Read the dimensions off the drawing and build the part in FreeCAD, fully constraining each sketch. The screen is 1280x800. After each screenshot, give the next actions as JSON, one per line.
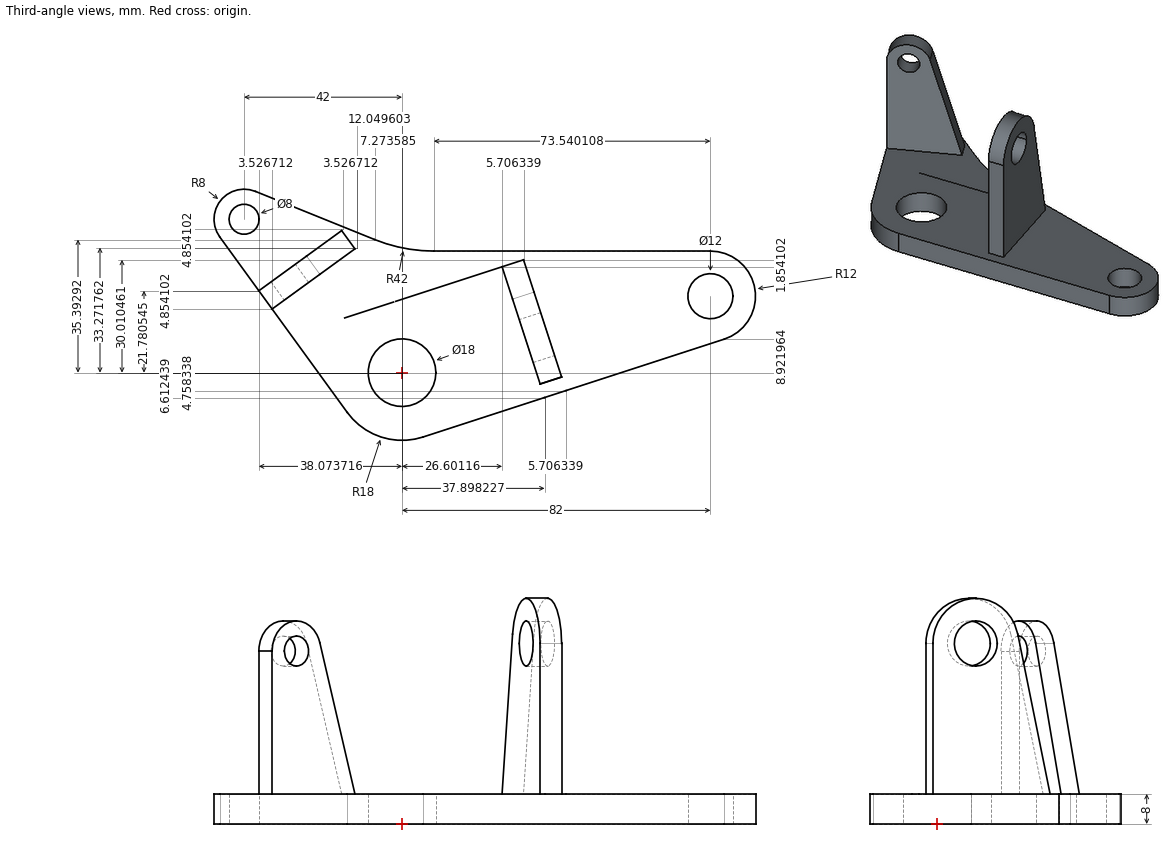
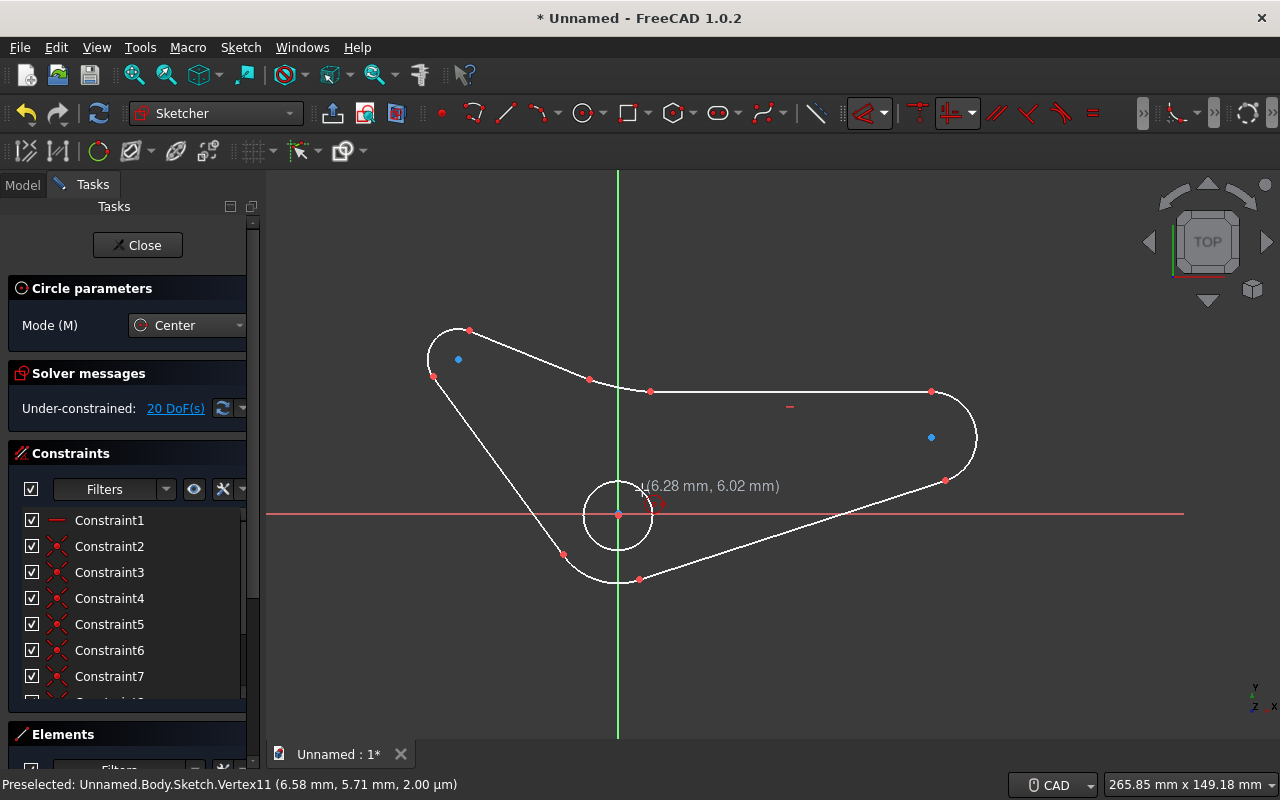
{"action": "scroll", "coordinate": [458, 358], "scroll_direction": "up", "scroll_amount": 2}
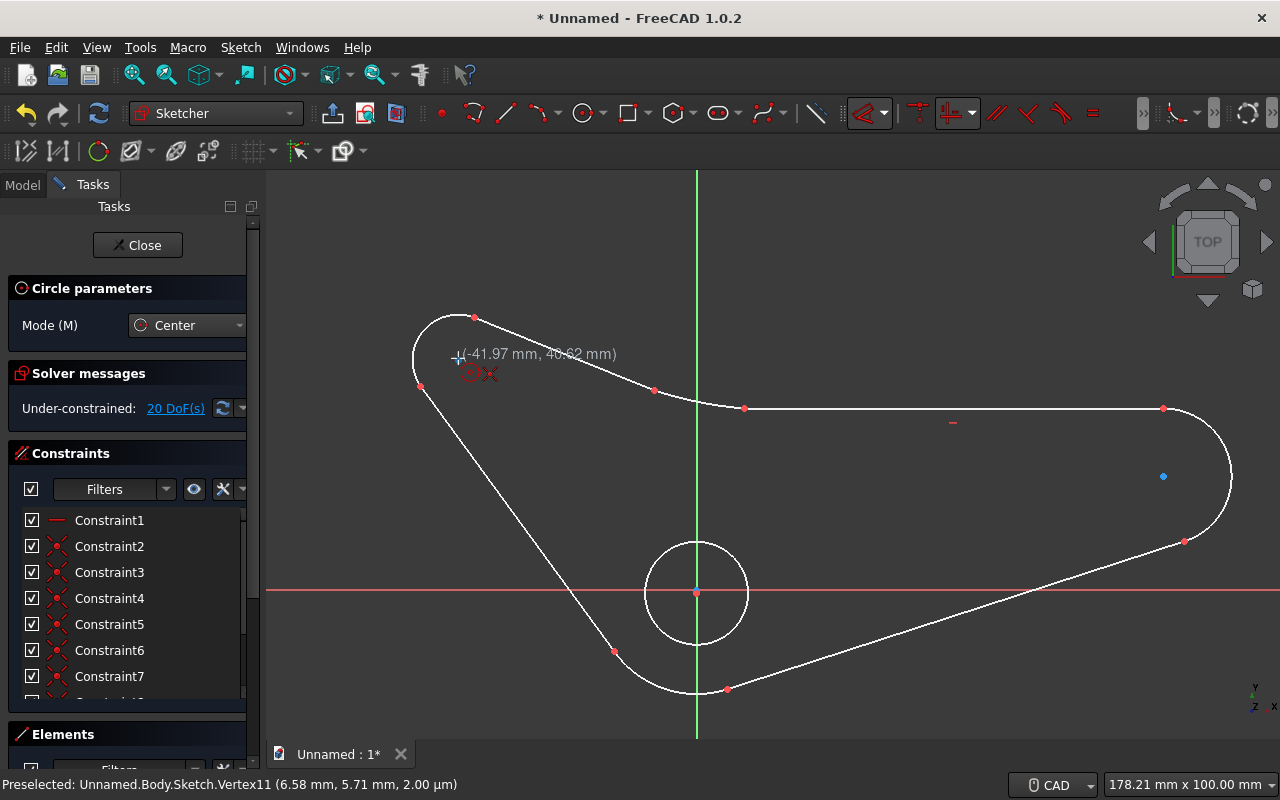
{"action": "left_click", "coordinate": [458, 358]}
{"action": "left_click", "coordinate": [474, 342]}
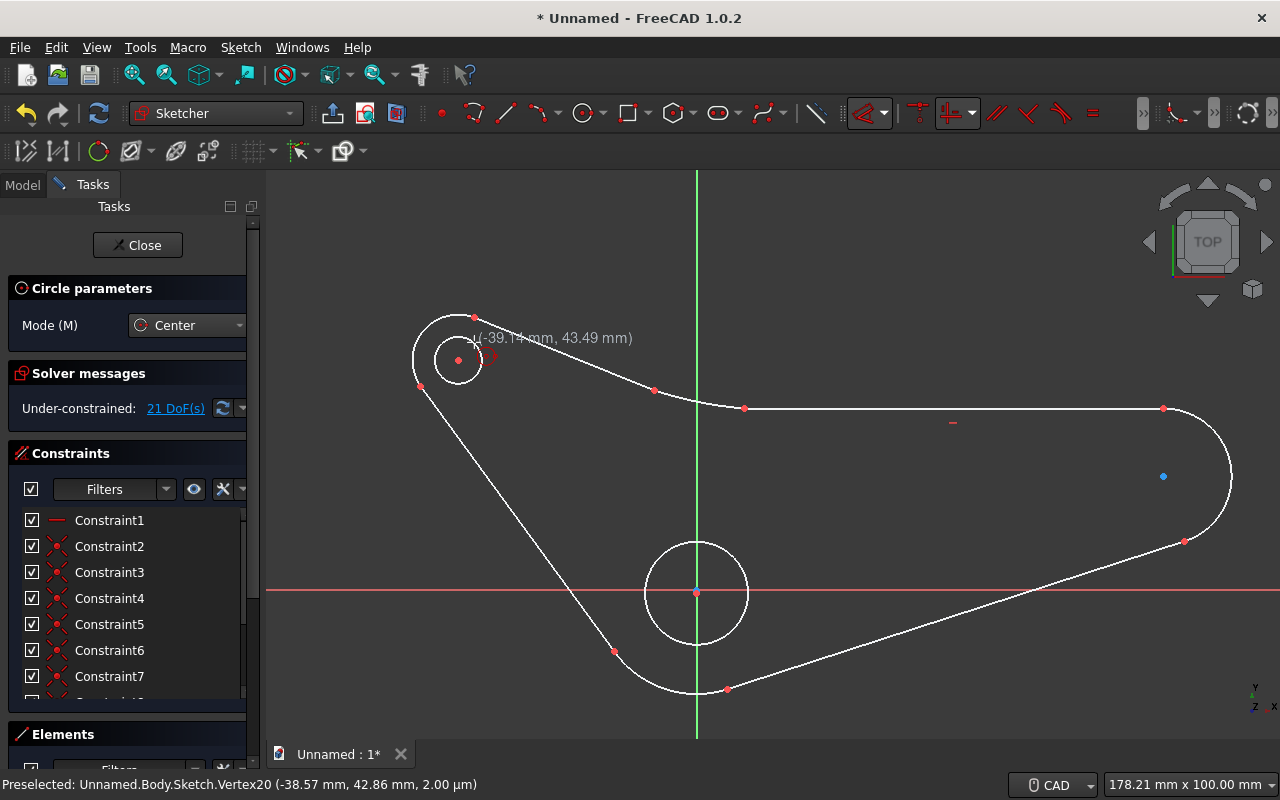
{"action": "scroll", "coordinate": [458, 358], "scroll_direction": "down", "scroll_amount": 2}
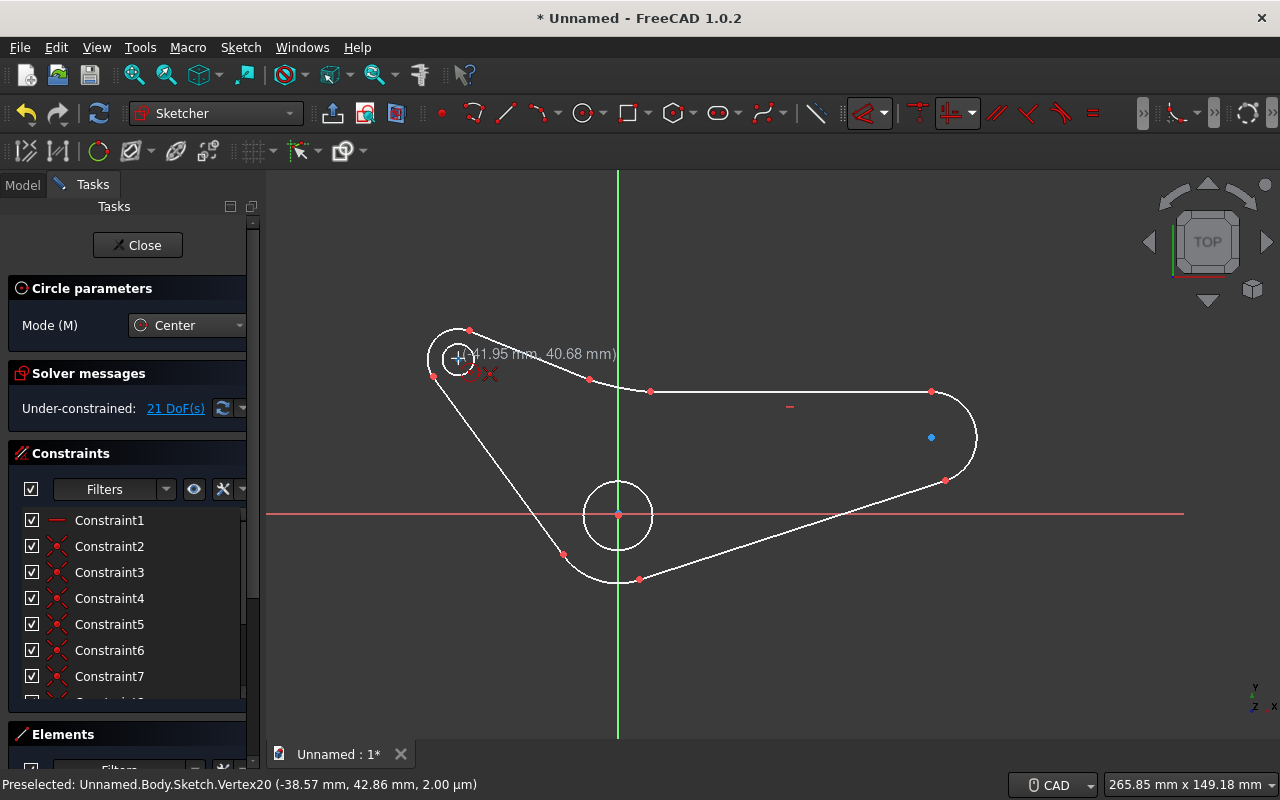
{"action": "left_click", "coordinate": [931, 436]}
{"action": "left_click", "coordinate": [947, 420]}
{"action": "key", "text": "Escape"}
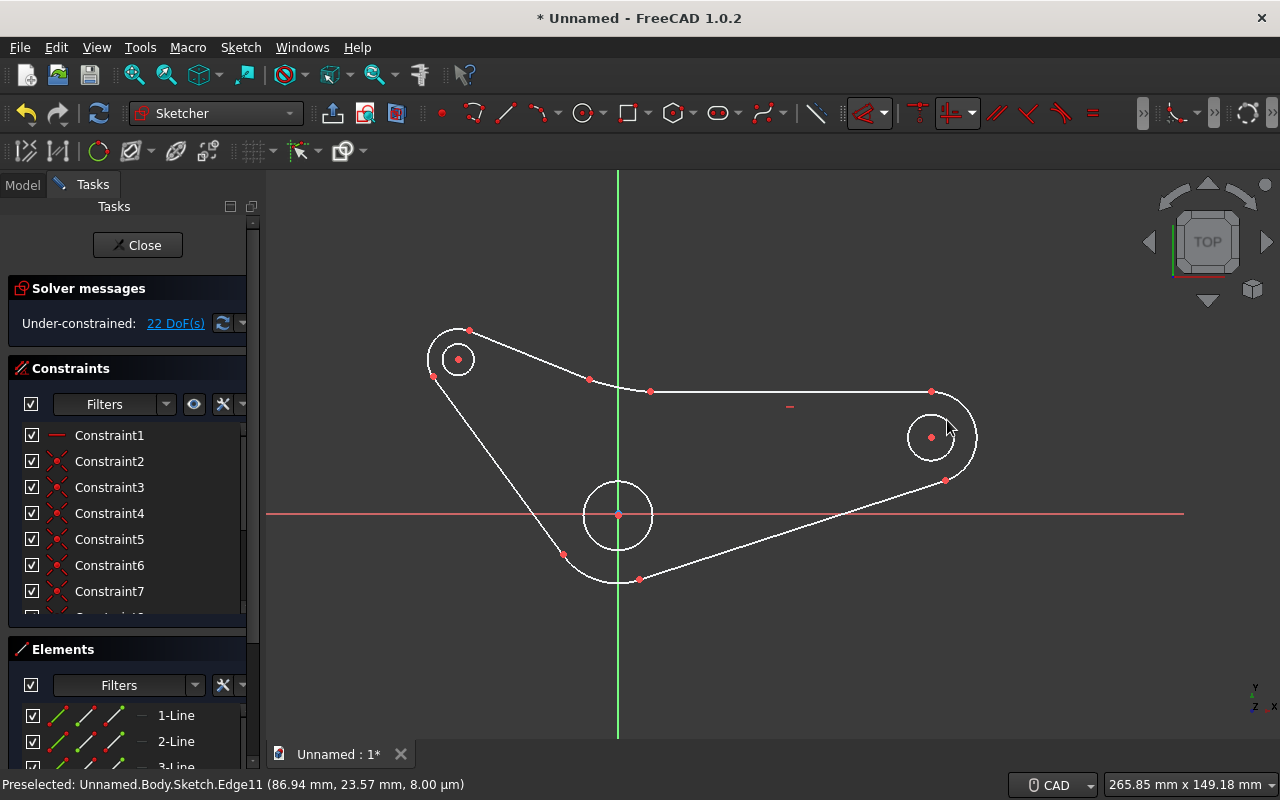
{"action": "left_click", "coordinate": [472, 430]}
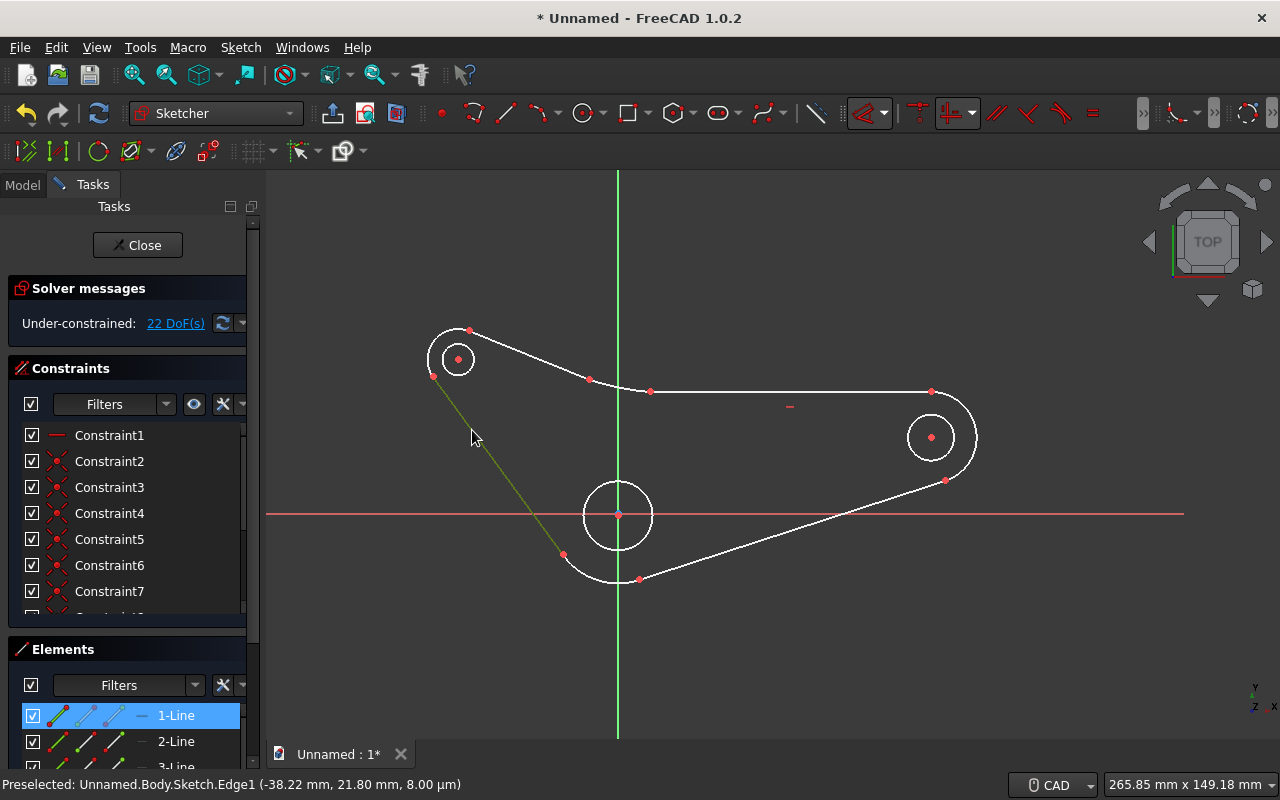
{"action": "left_click", "coordinate": [581, 573]}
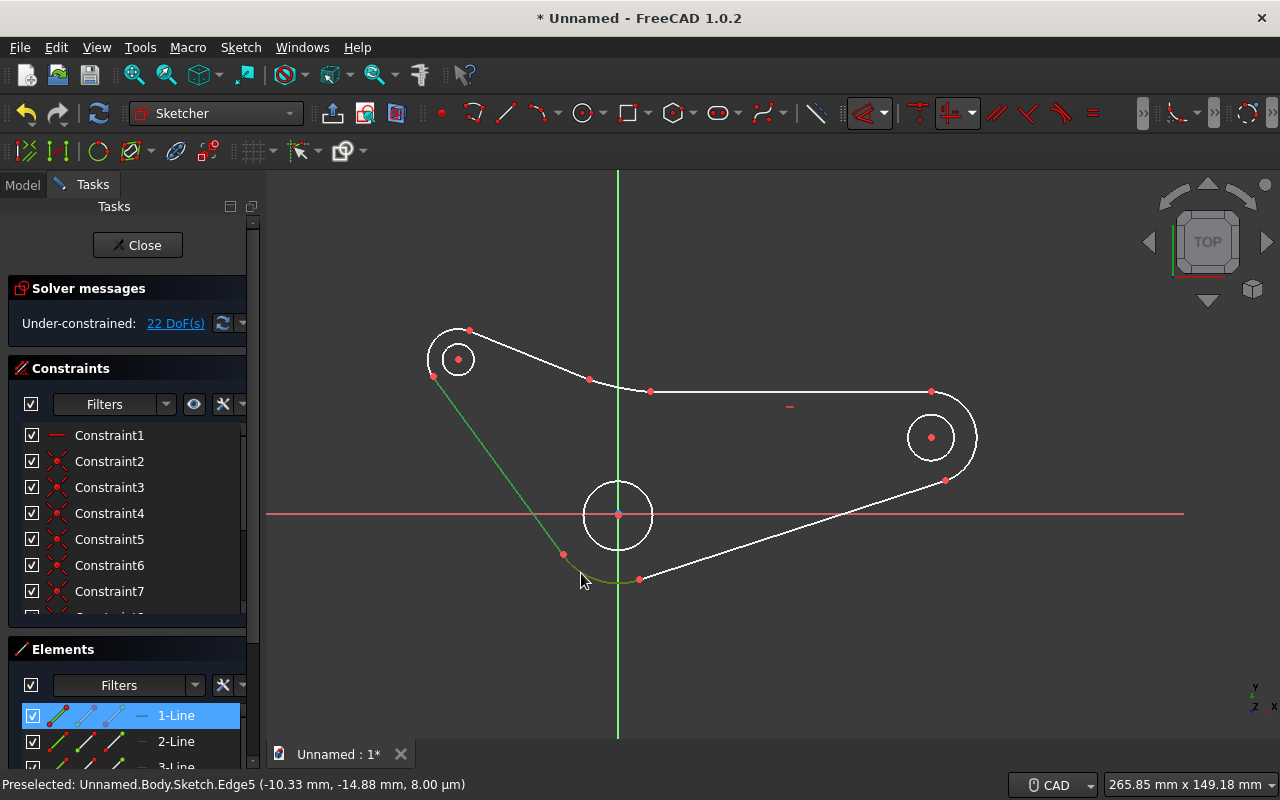
{"action": "key", "text": "t"}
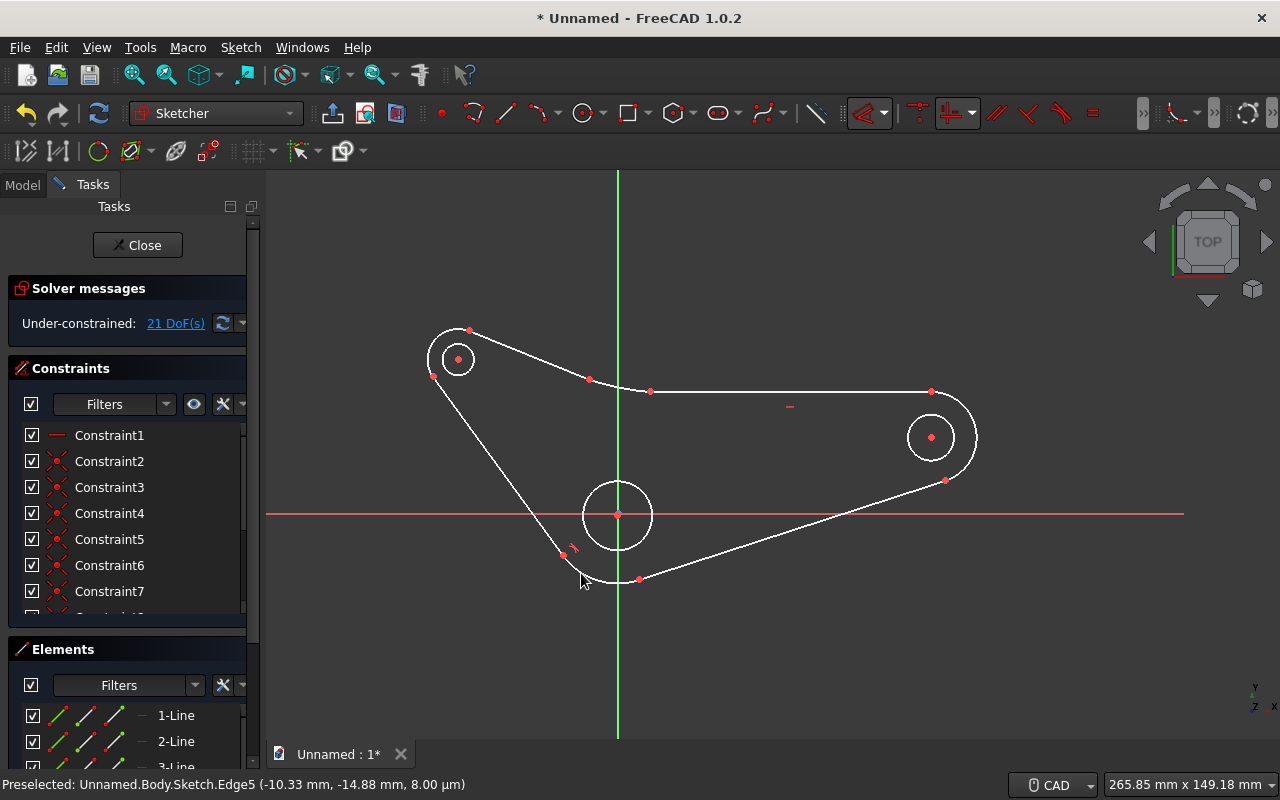
{"action": "left_click", "coordinate": [472, 431]}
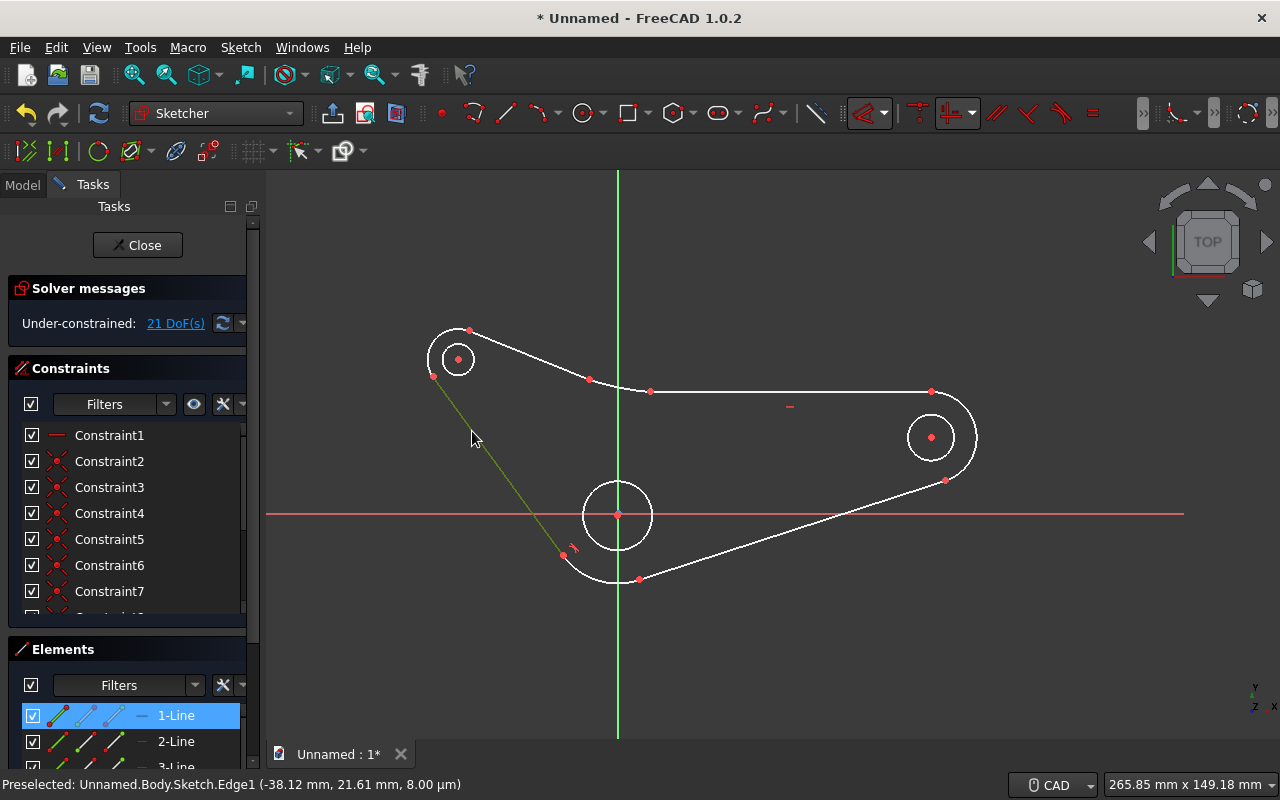
{"action": "left_click", "coordinate": [446, 331]}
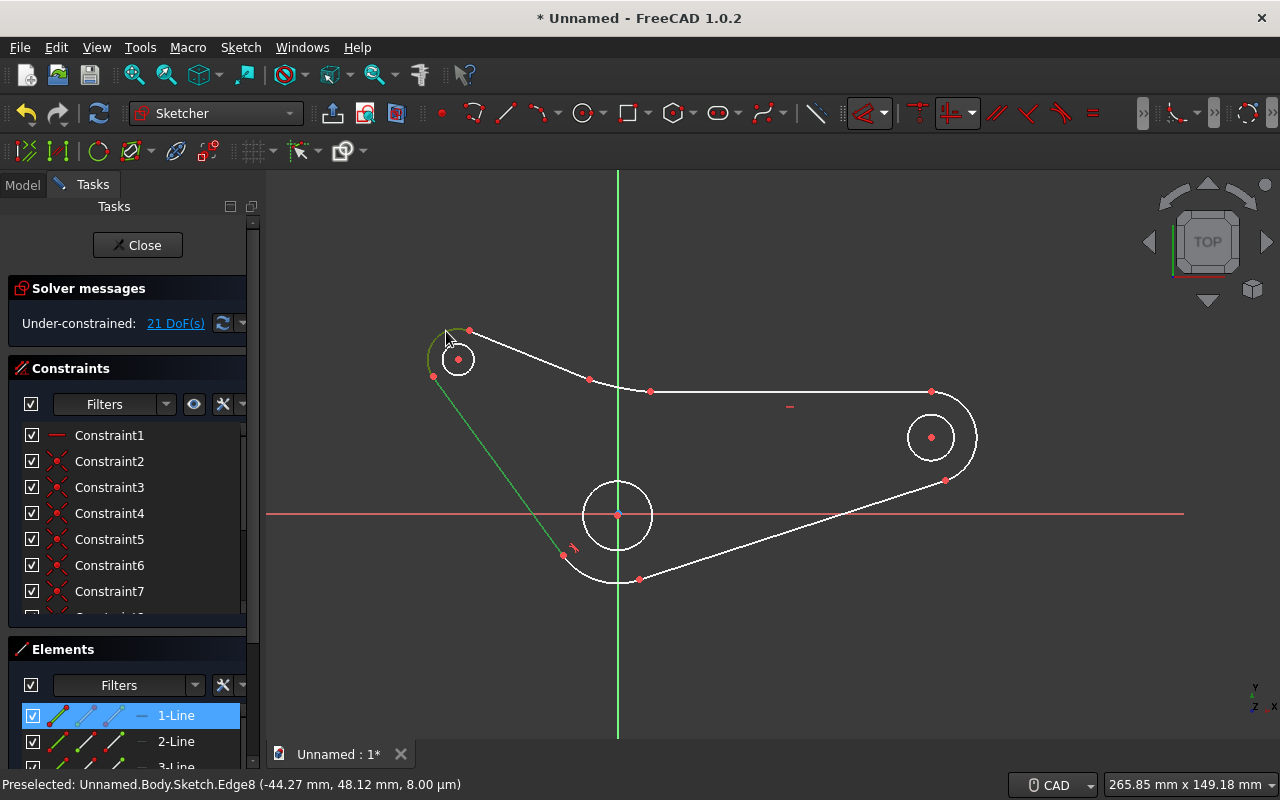
{"action": "key", "text": "t"}